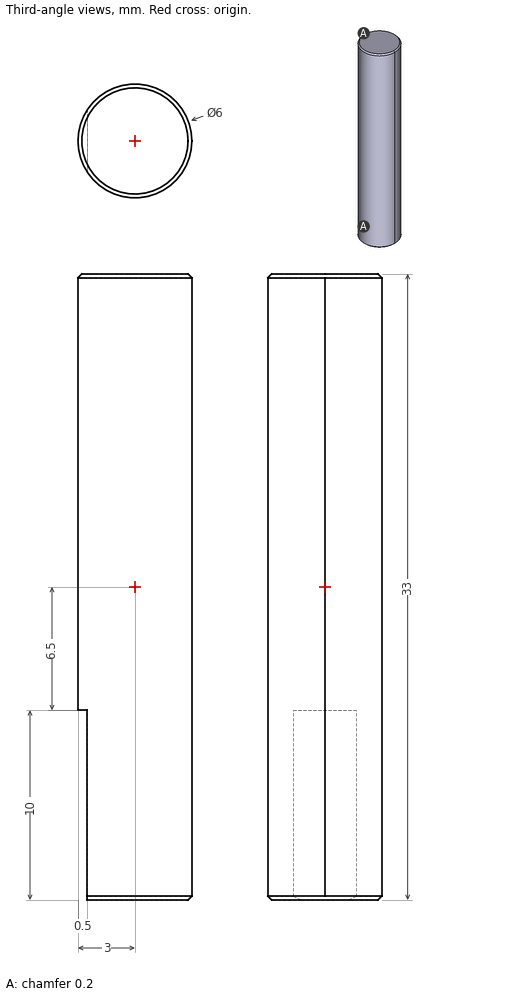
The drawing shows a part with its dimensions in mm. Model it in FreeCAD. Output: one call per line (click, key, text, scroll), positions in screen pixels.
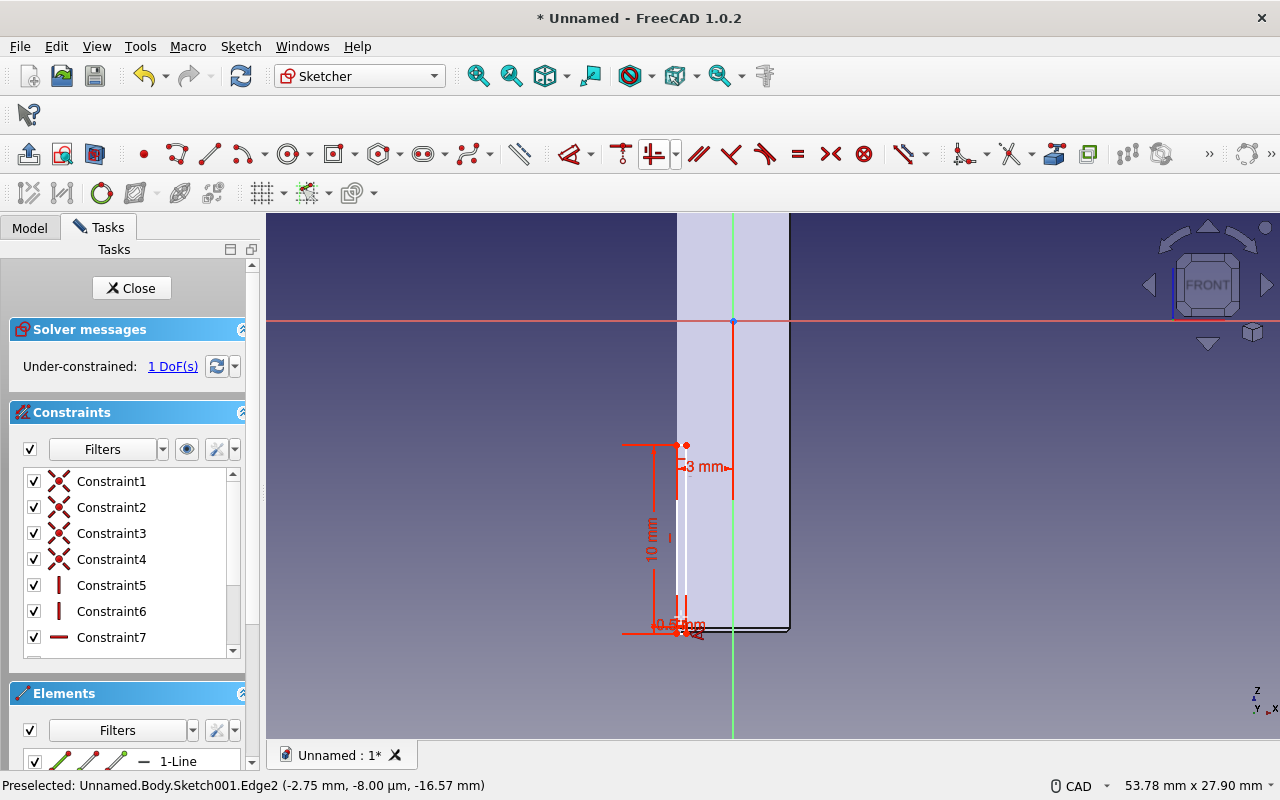
scroll(677, 445, up, 2)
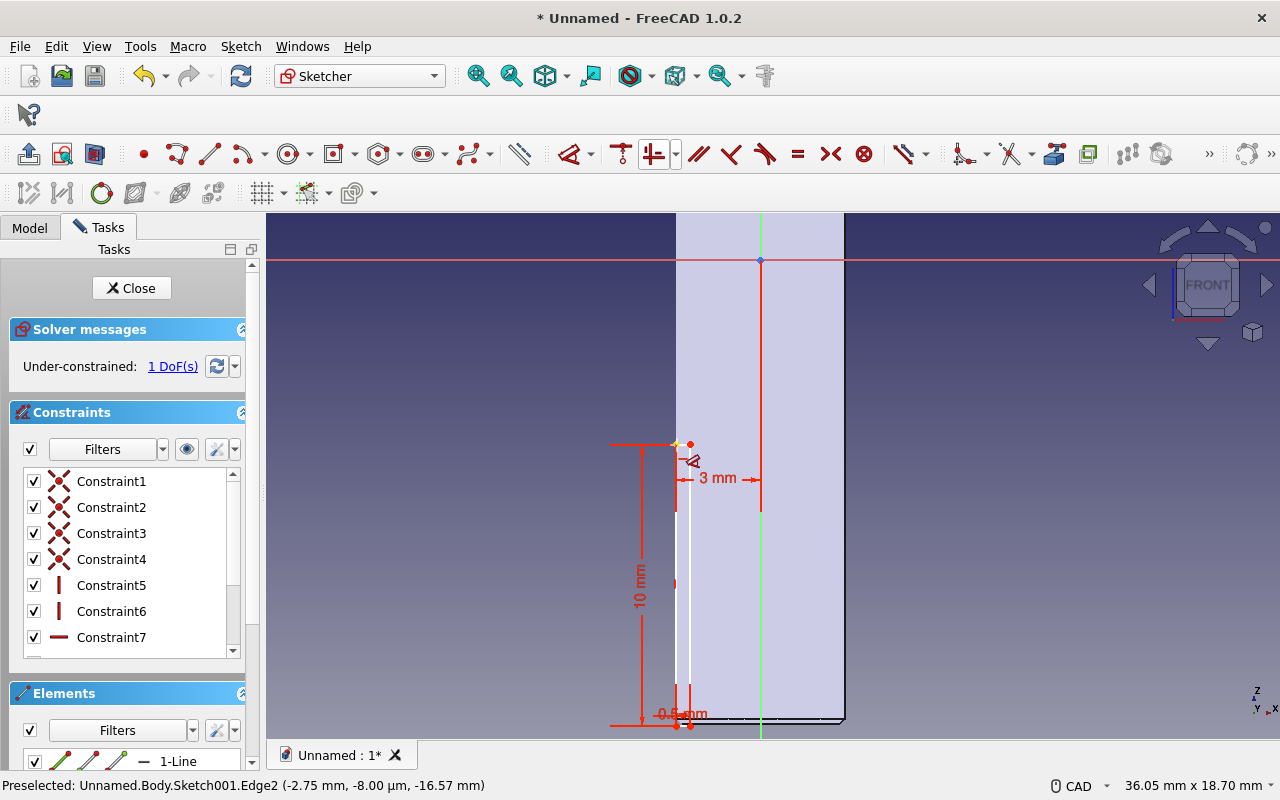
click(676, 445)
click(795, 352)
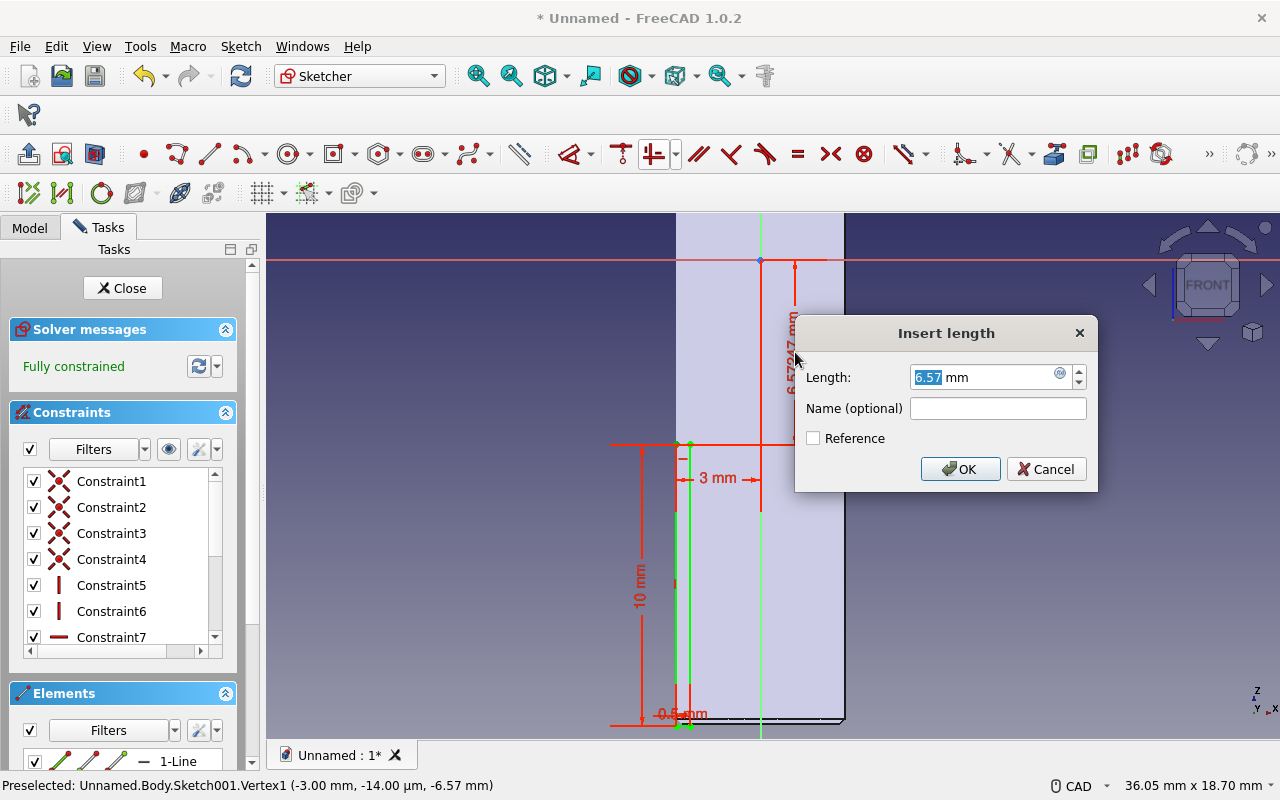
text(6.5)
key(Return)
key(Escape)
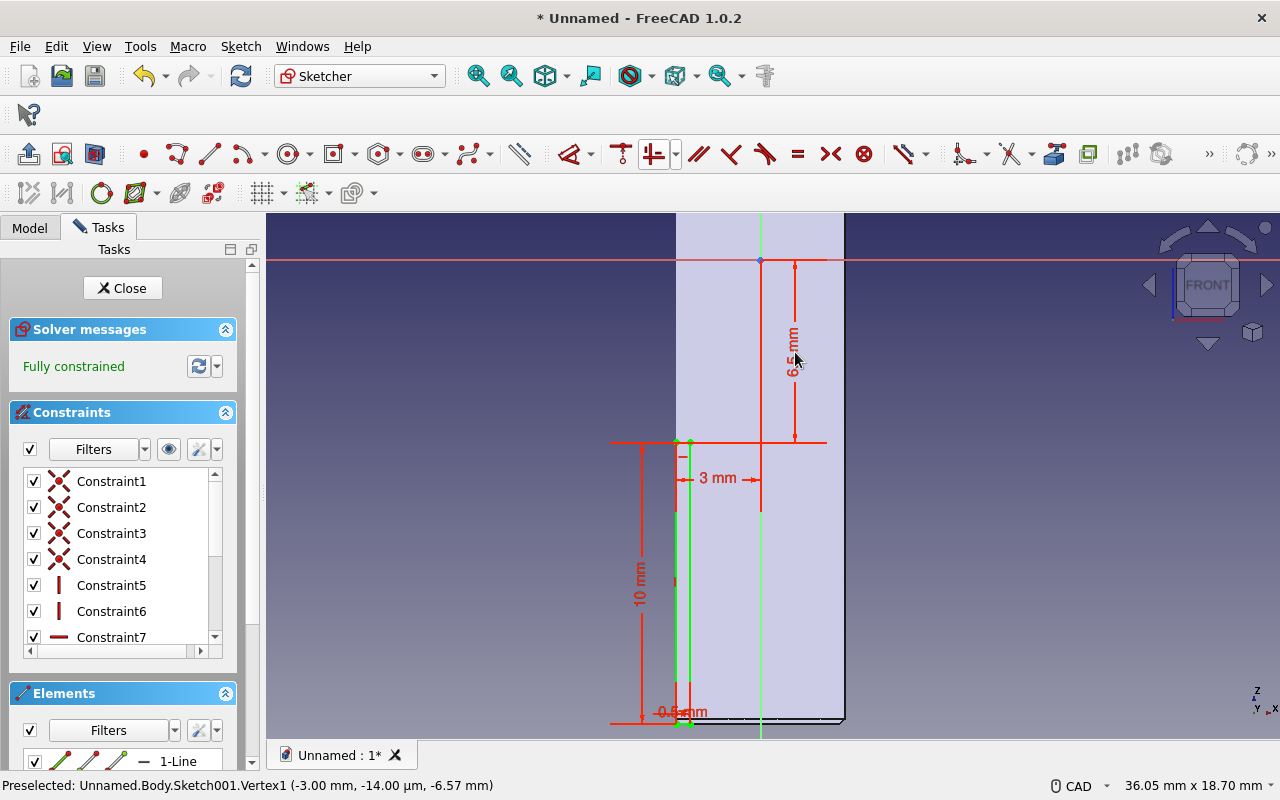
click(123, 288)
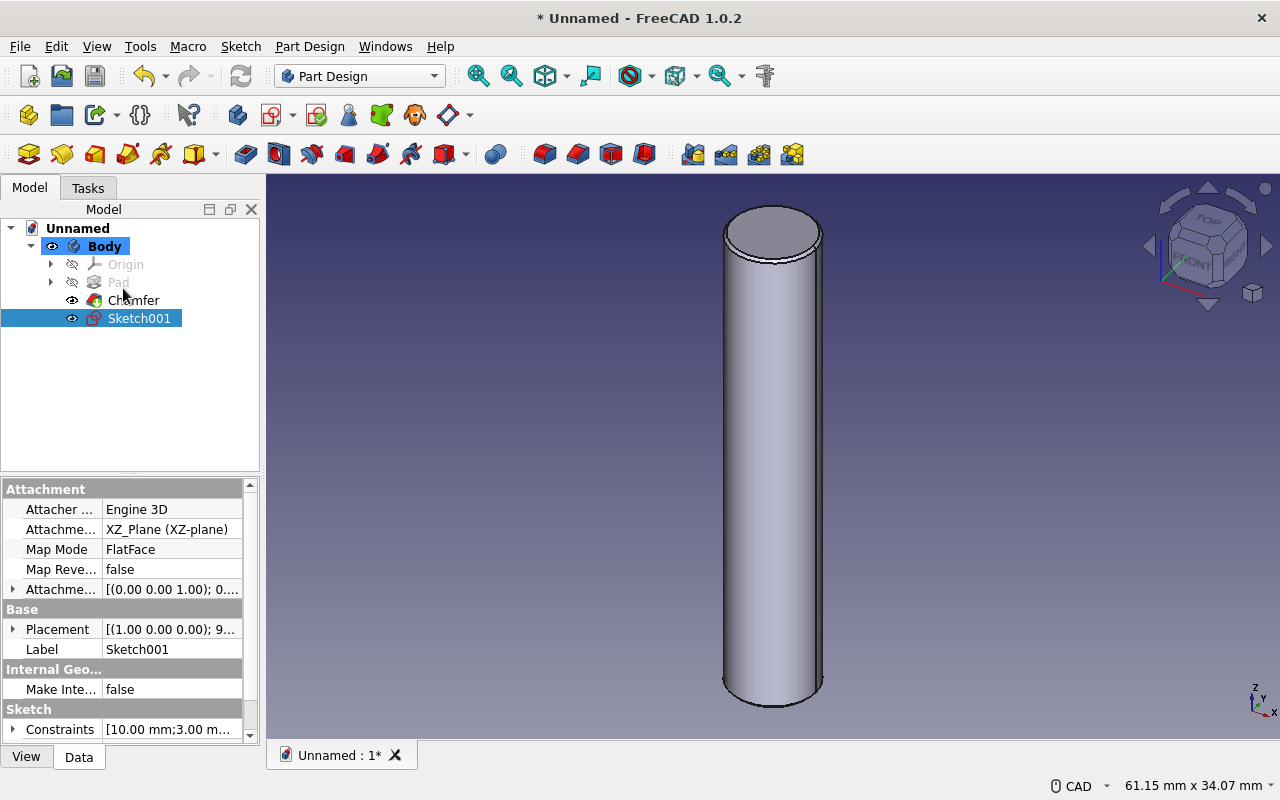
click(246, 154)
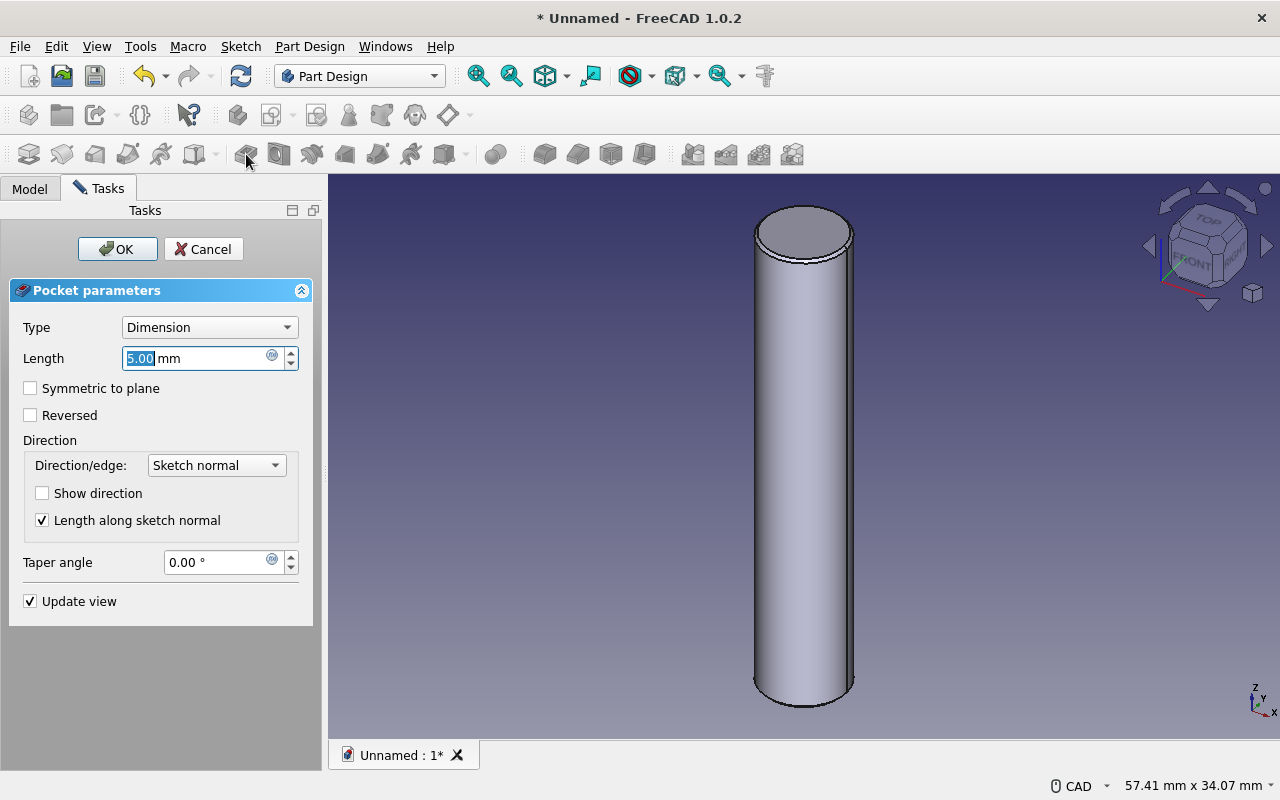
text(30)
key(Tab)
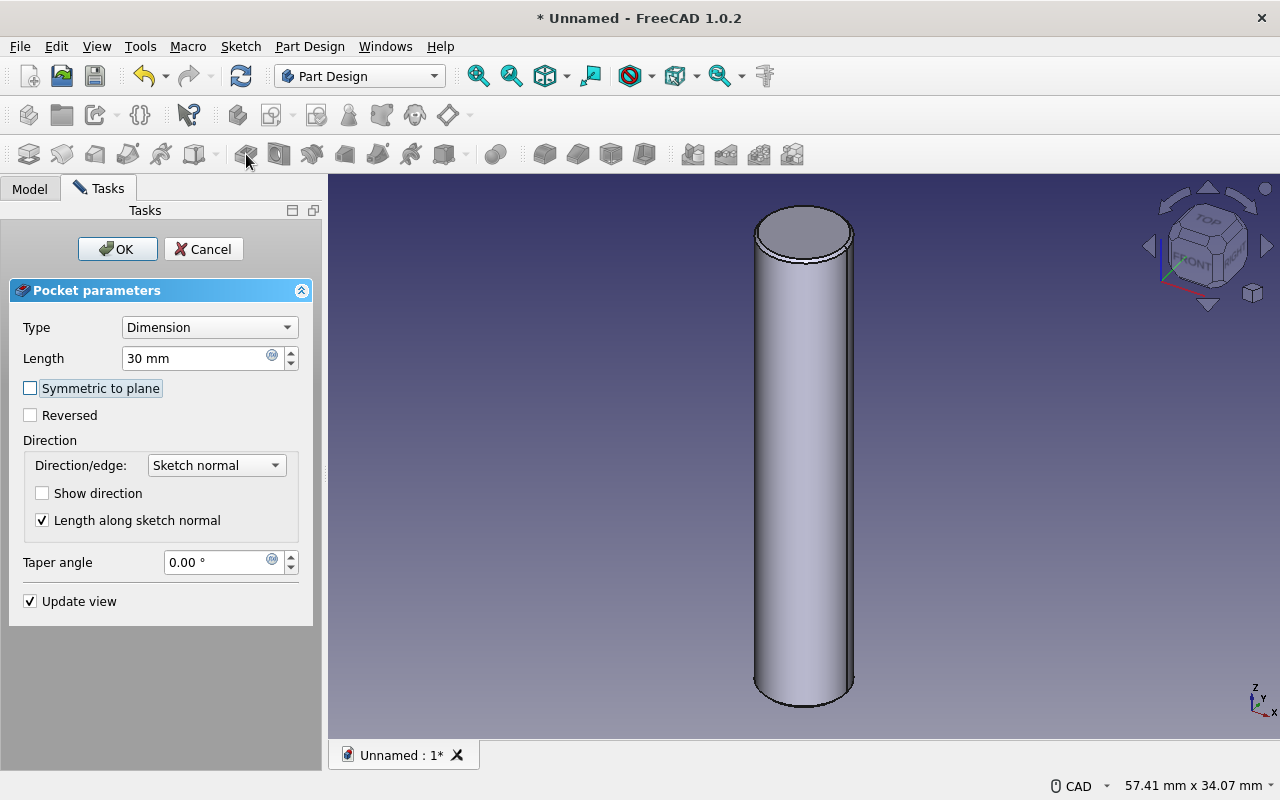
click(31, 388)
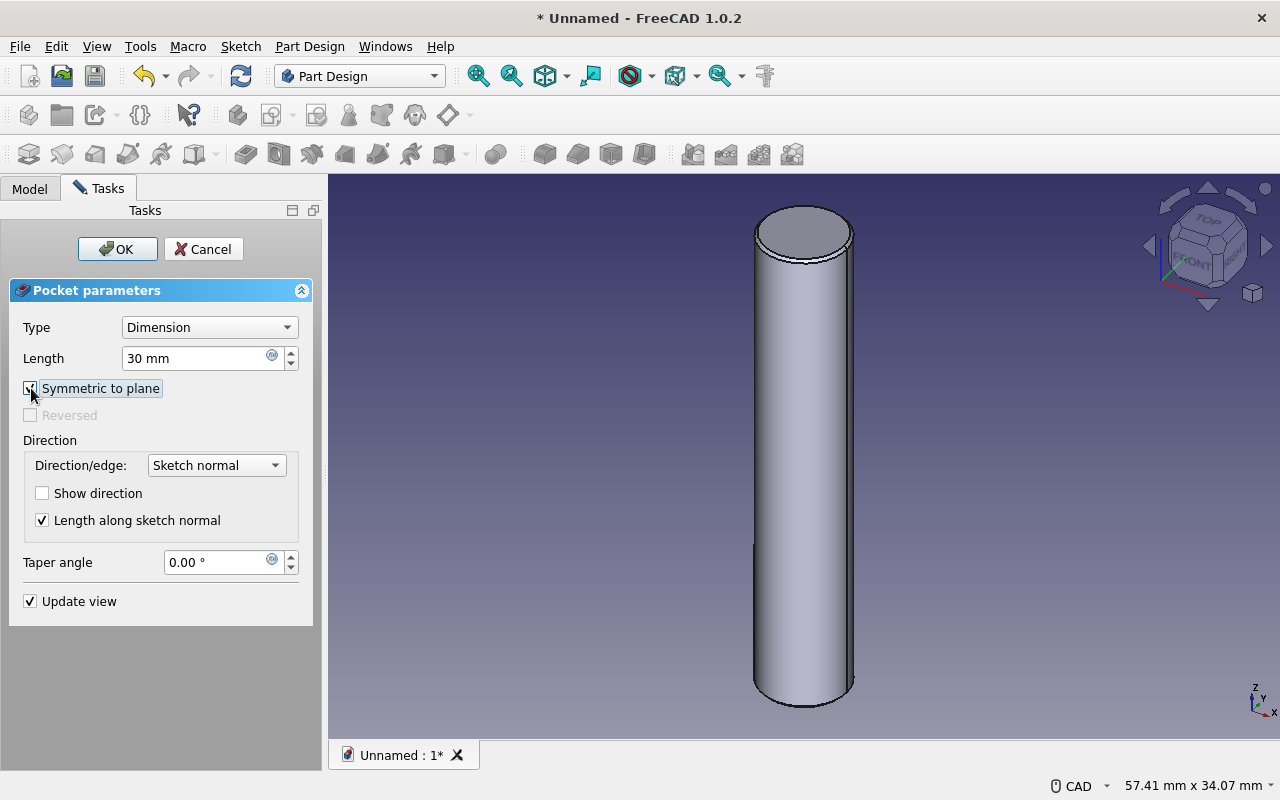
click(118, 249)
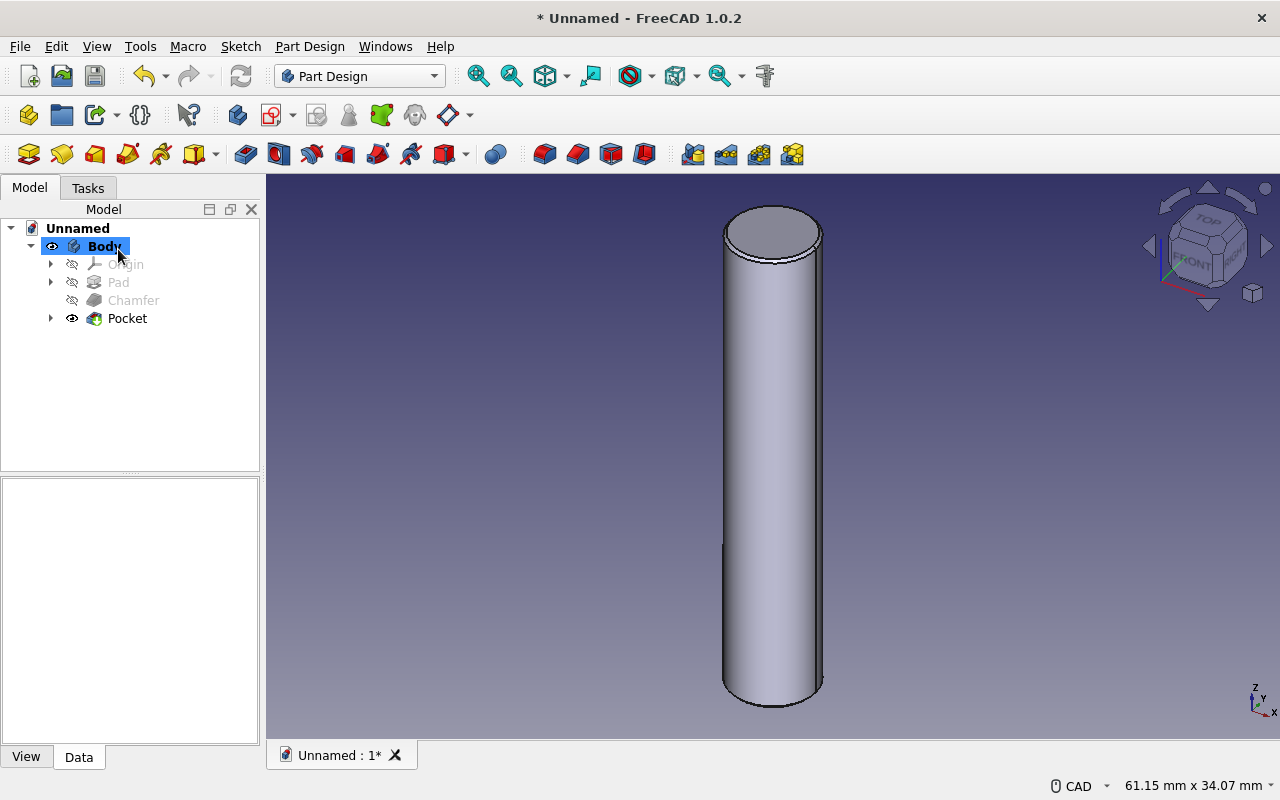
key(0)